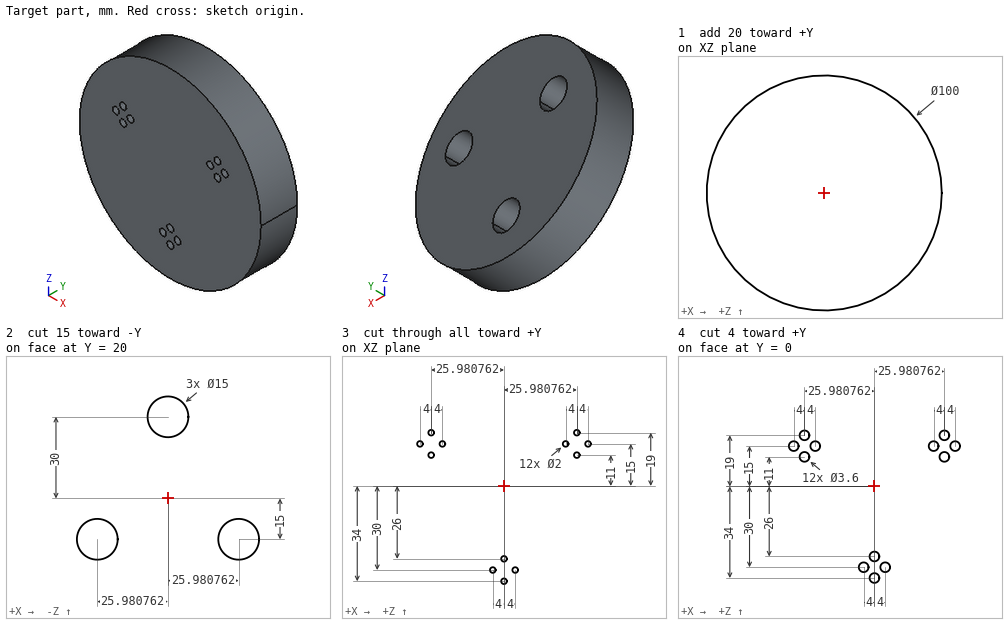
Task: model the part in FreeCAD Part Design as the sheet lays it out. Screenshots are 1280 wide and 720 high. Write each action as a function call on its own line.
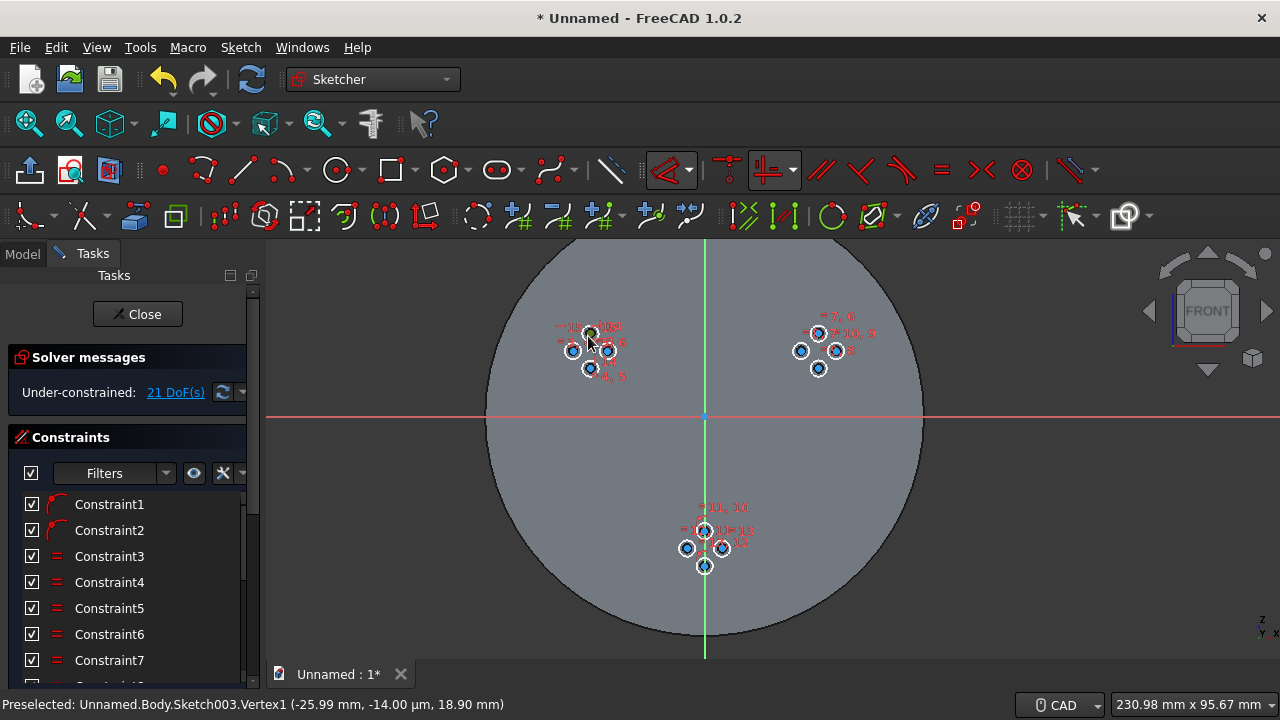
click(819, 334)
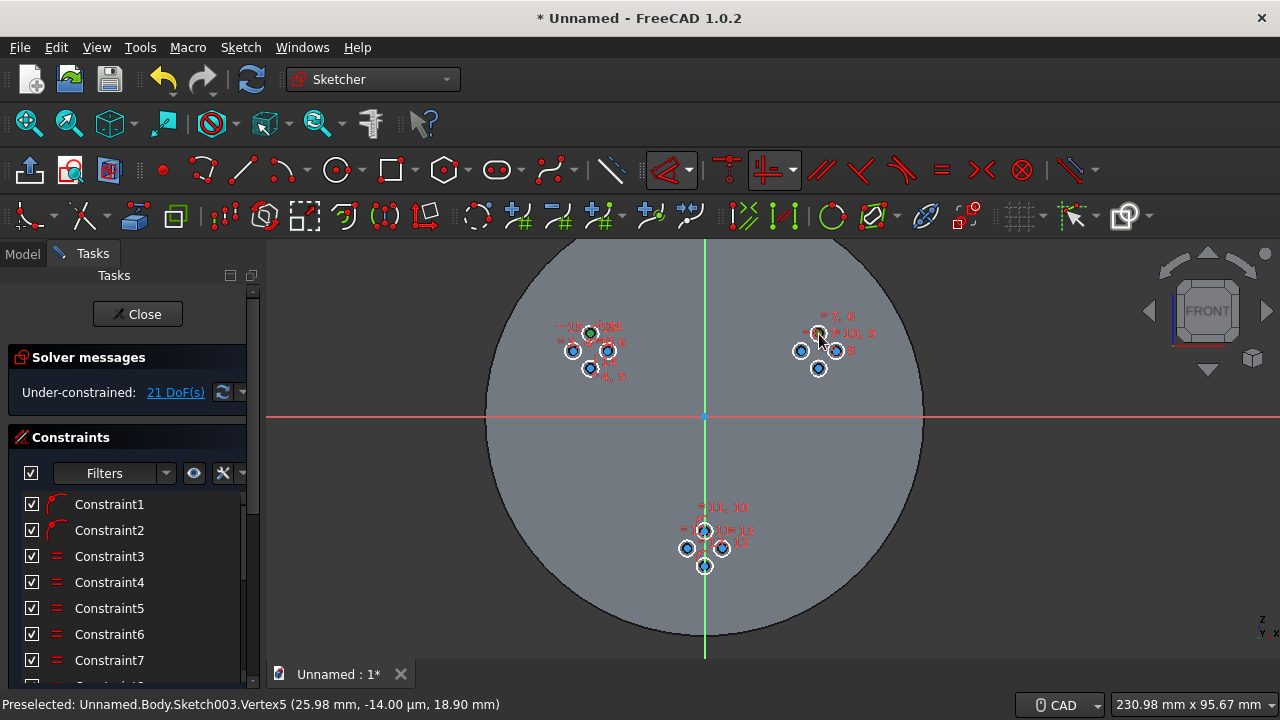
click(796, 170)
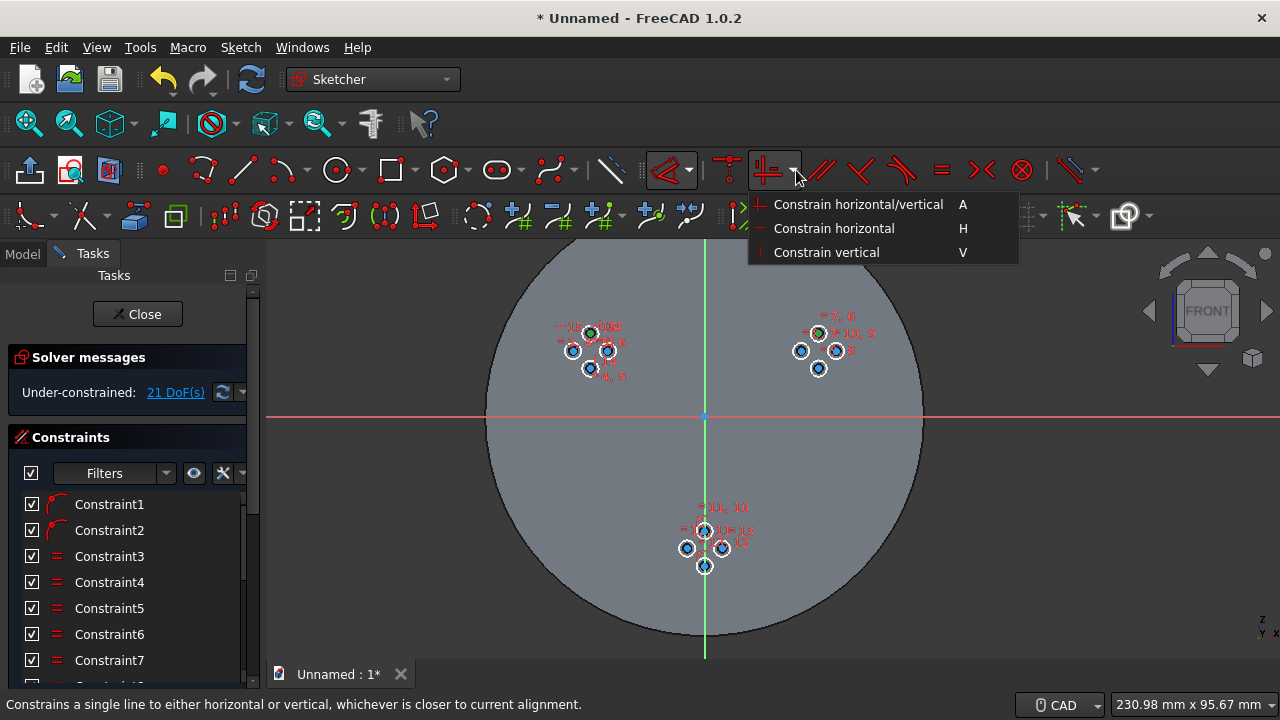
click(884, 228)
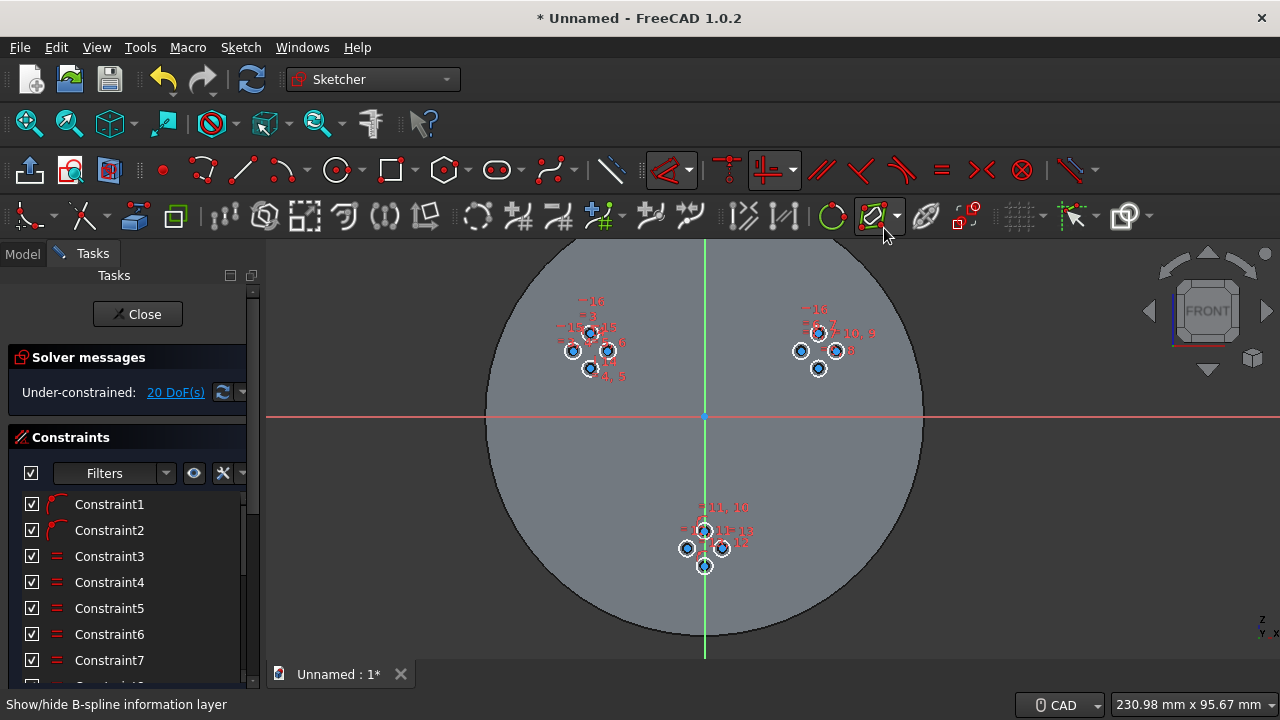
click(608, 351)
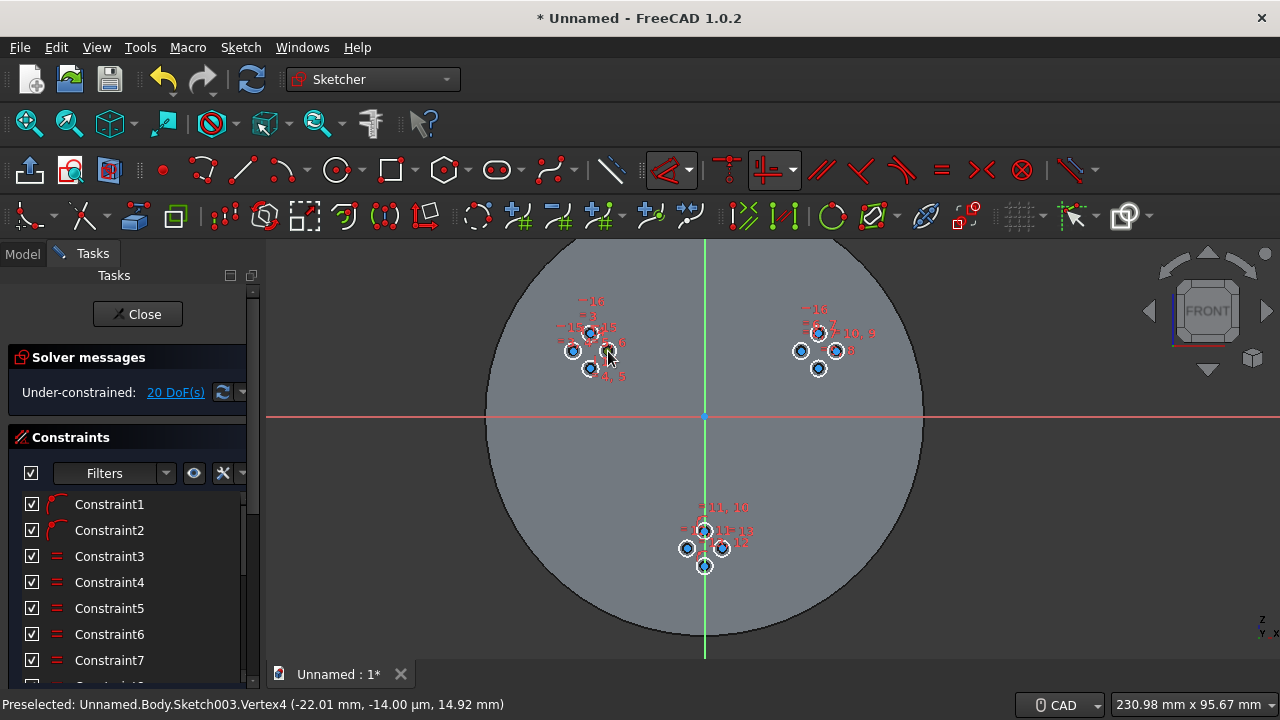
click(801, 351)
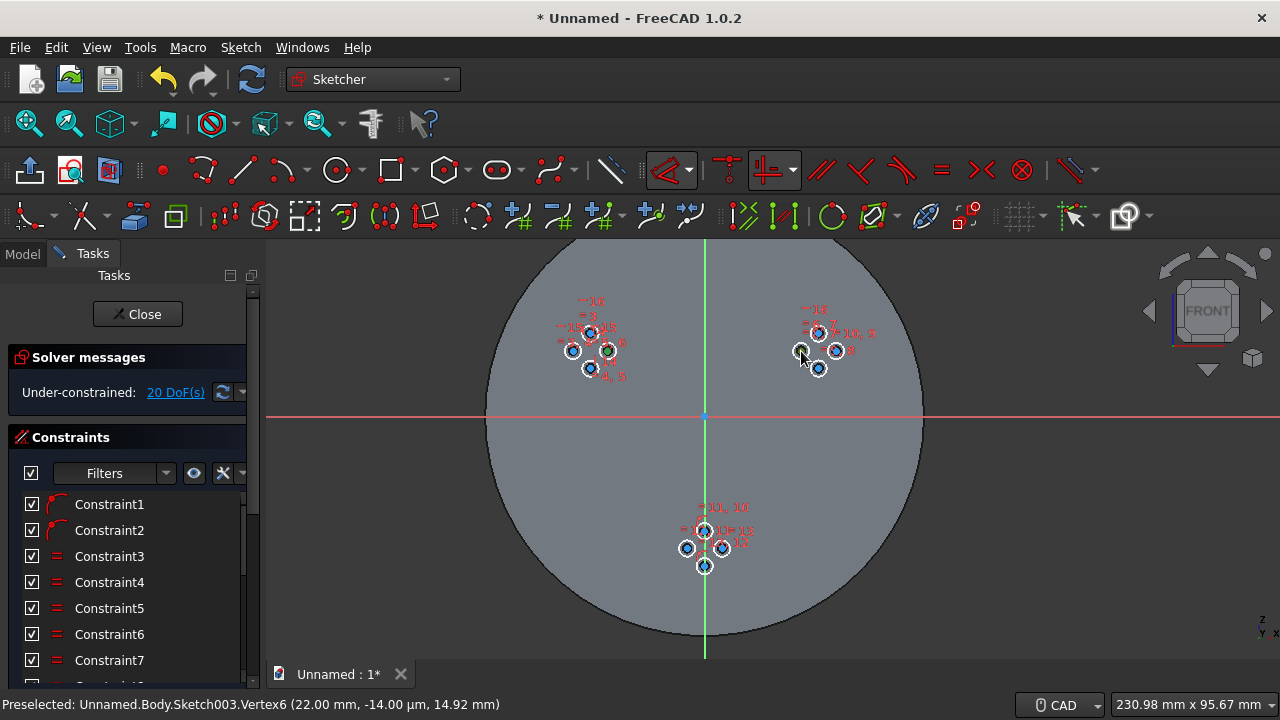
click(796, 170)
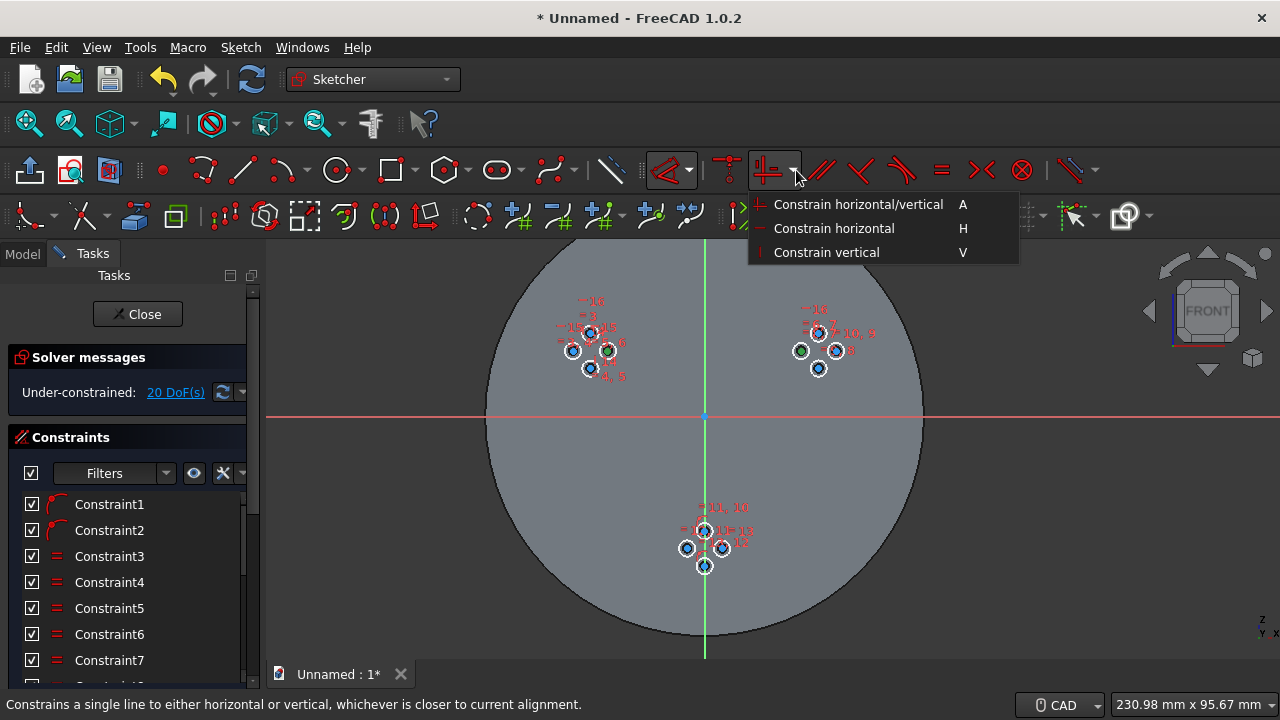
click(884, 228)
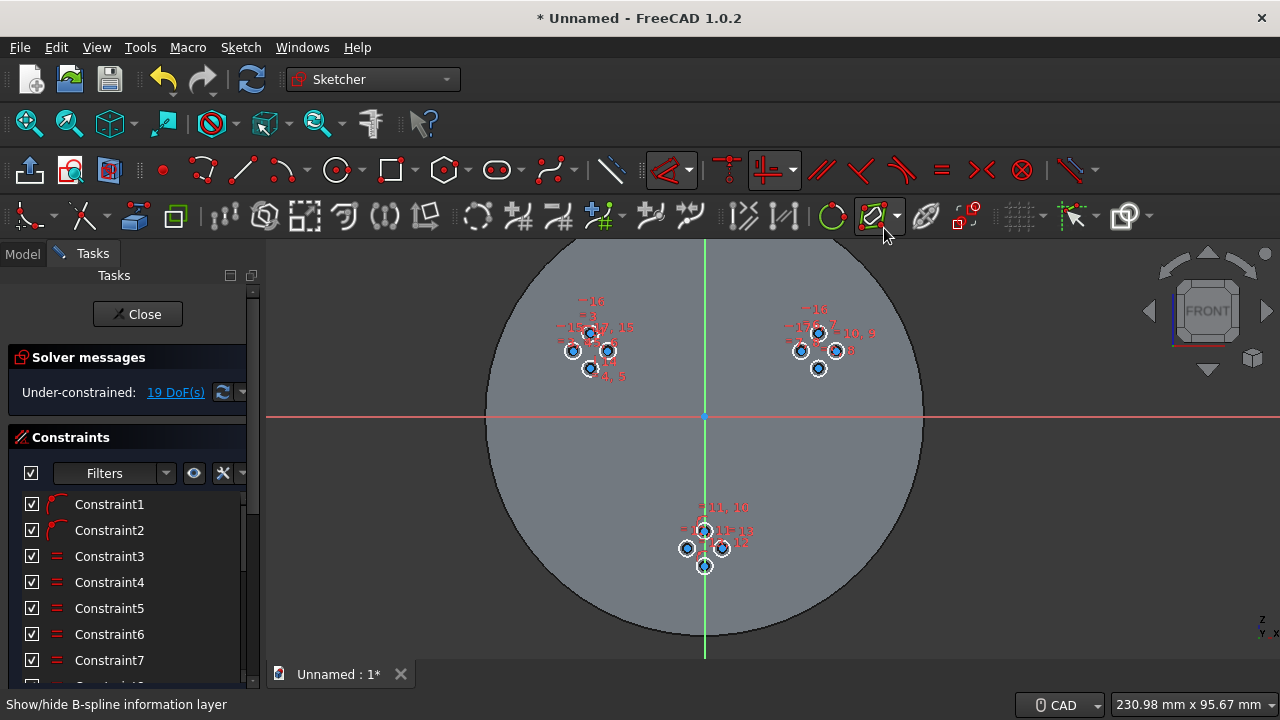
click(821, 336)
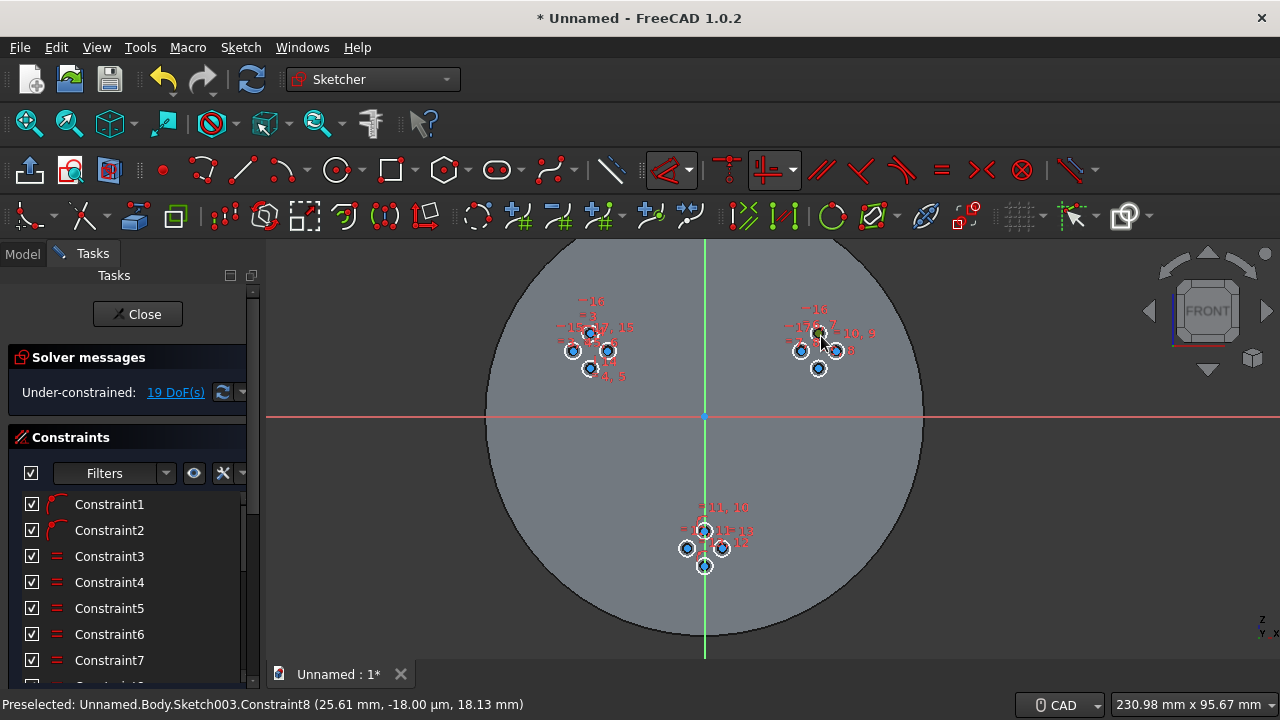
click(819, 369)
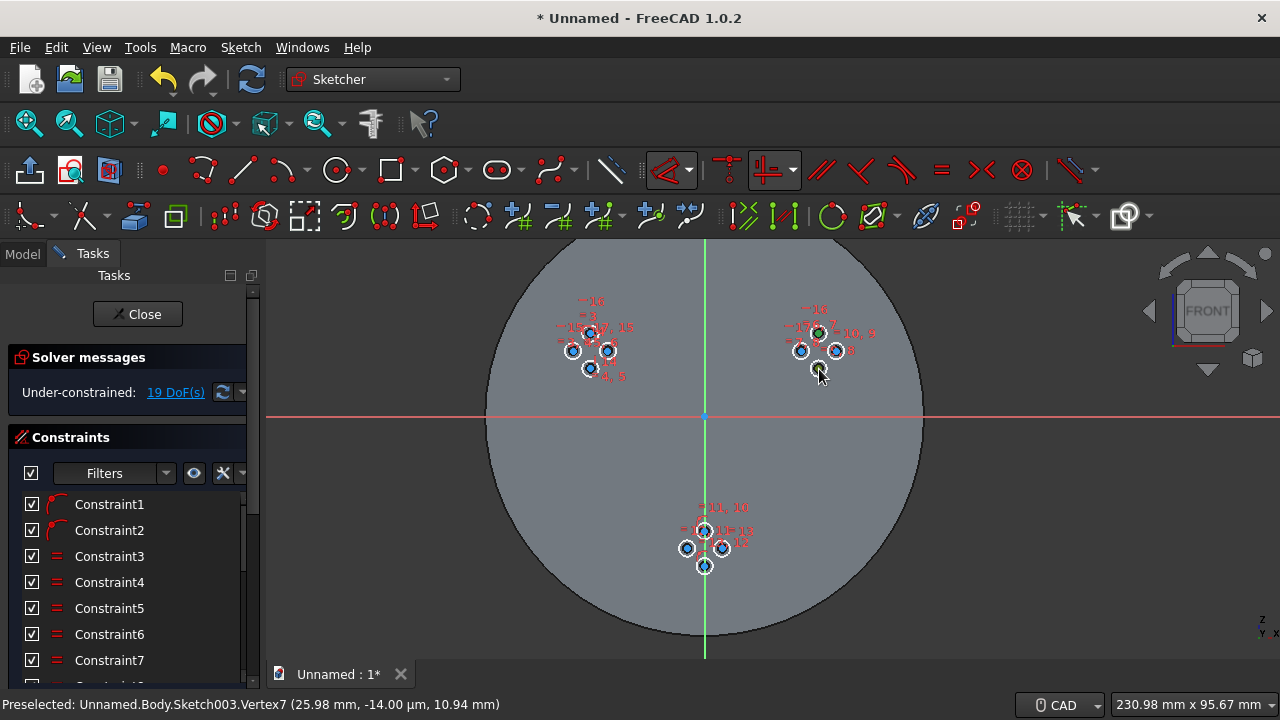
click(796, 170)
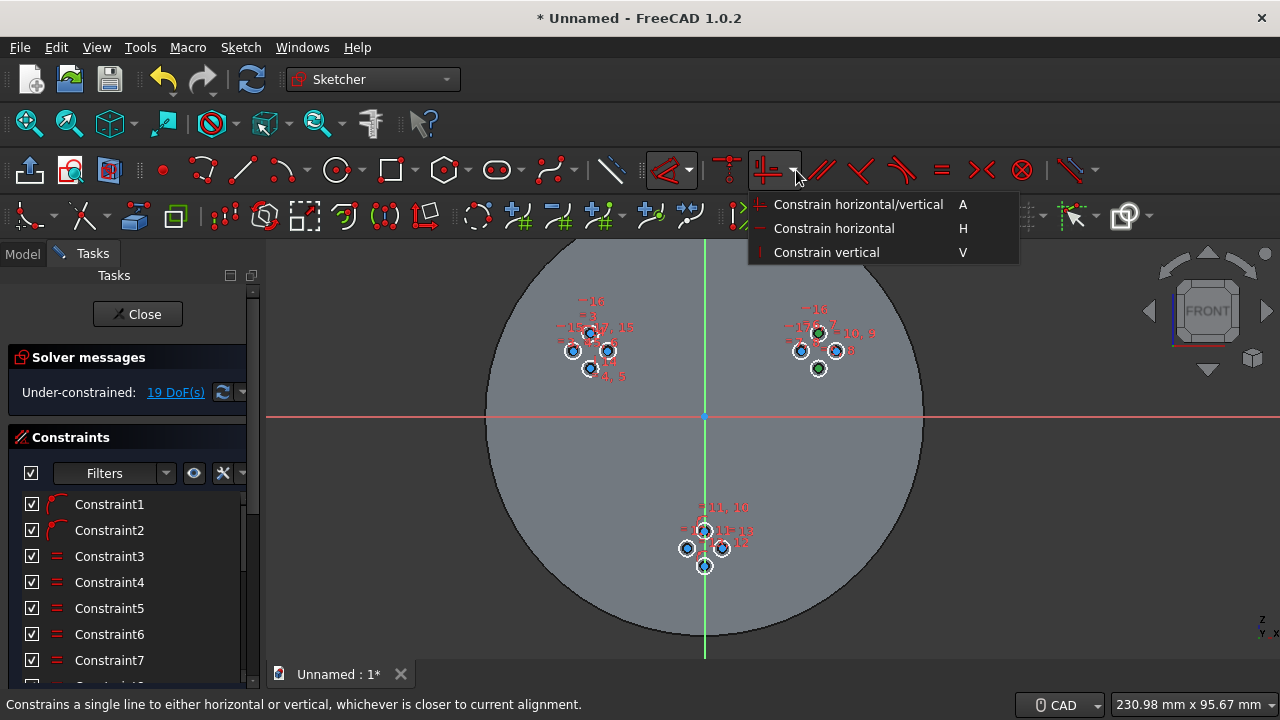
click(884, 252)